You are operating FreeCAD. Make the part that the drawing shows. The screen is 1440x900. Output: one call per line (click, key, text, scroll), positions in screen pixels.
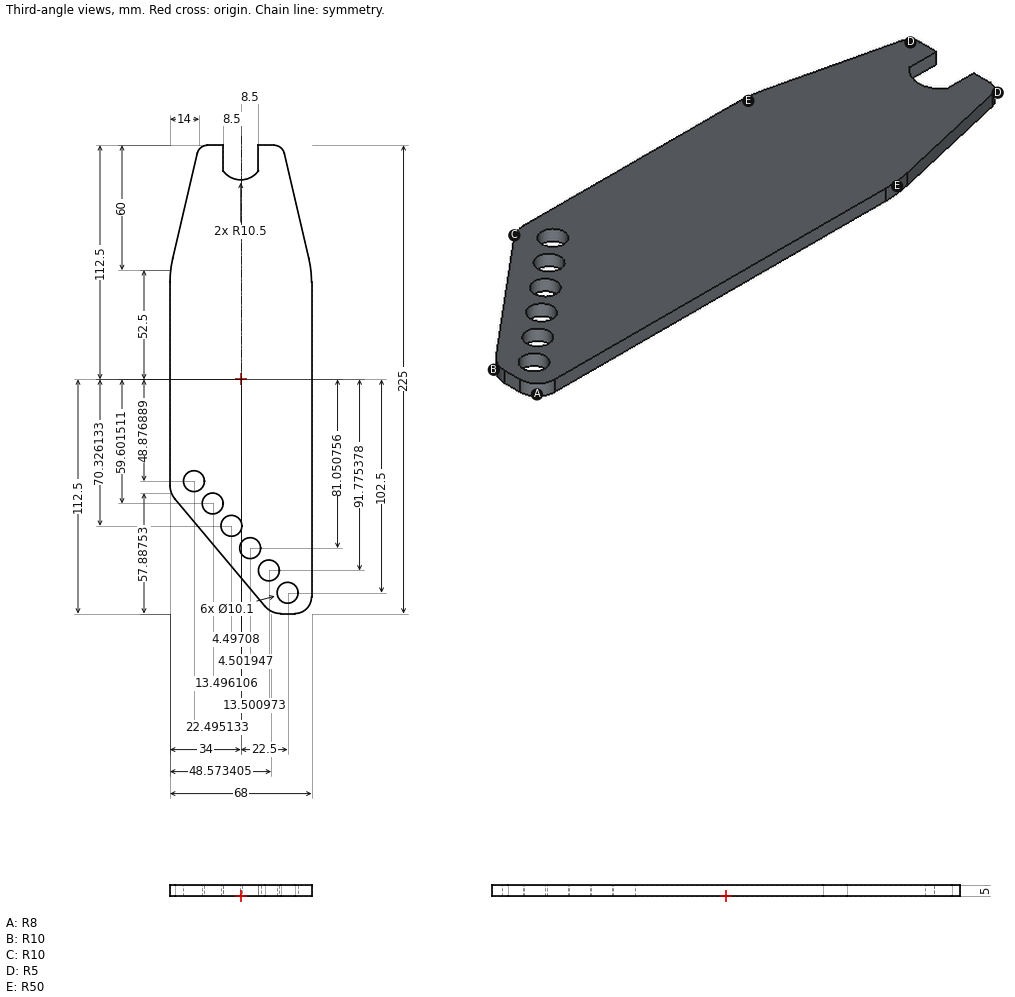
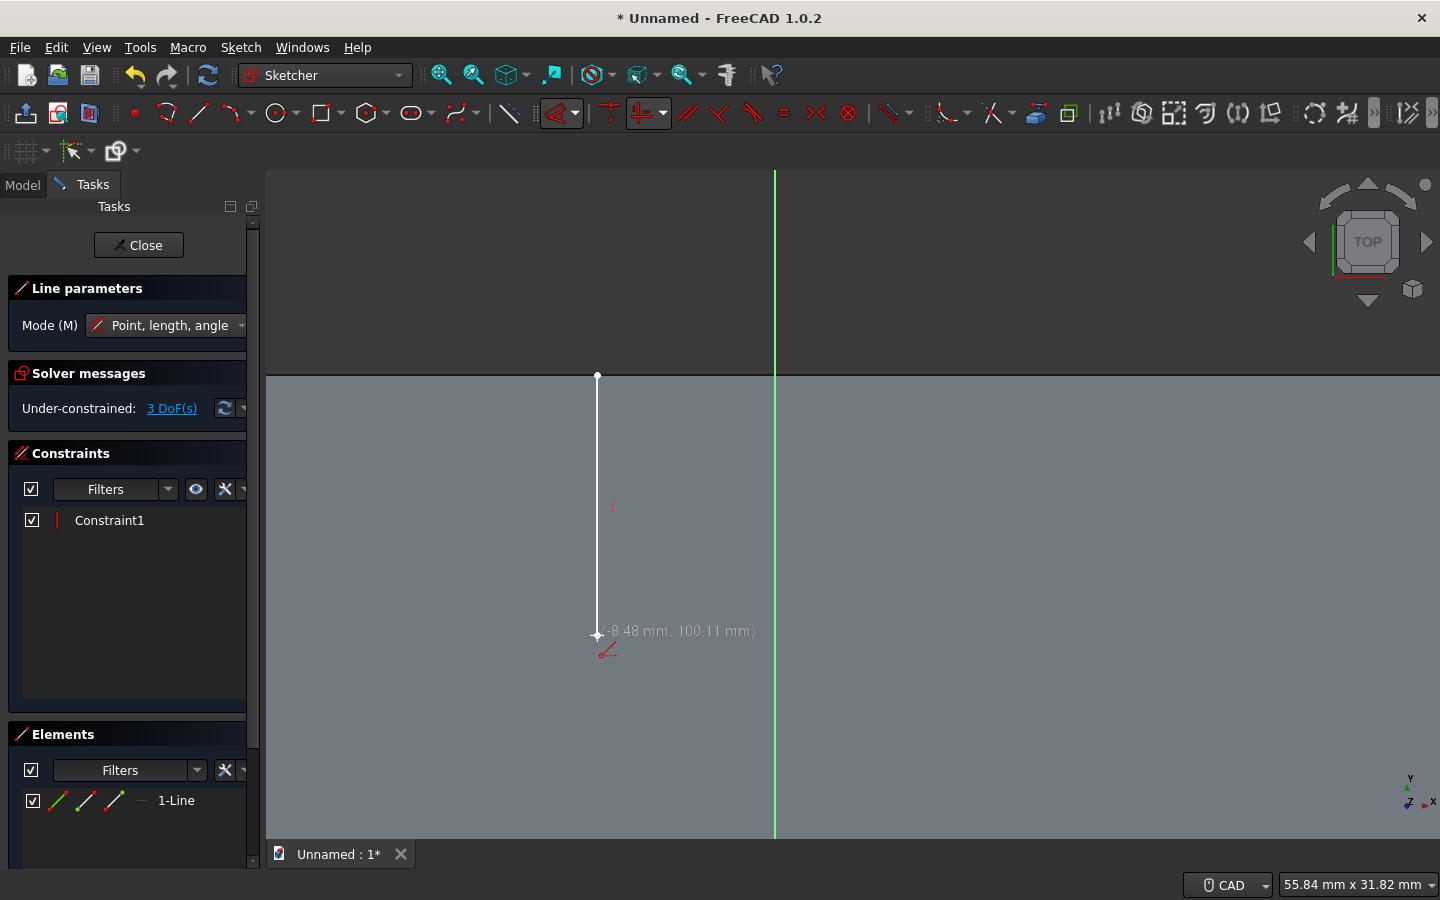
click(954, 635)
click(954, 375)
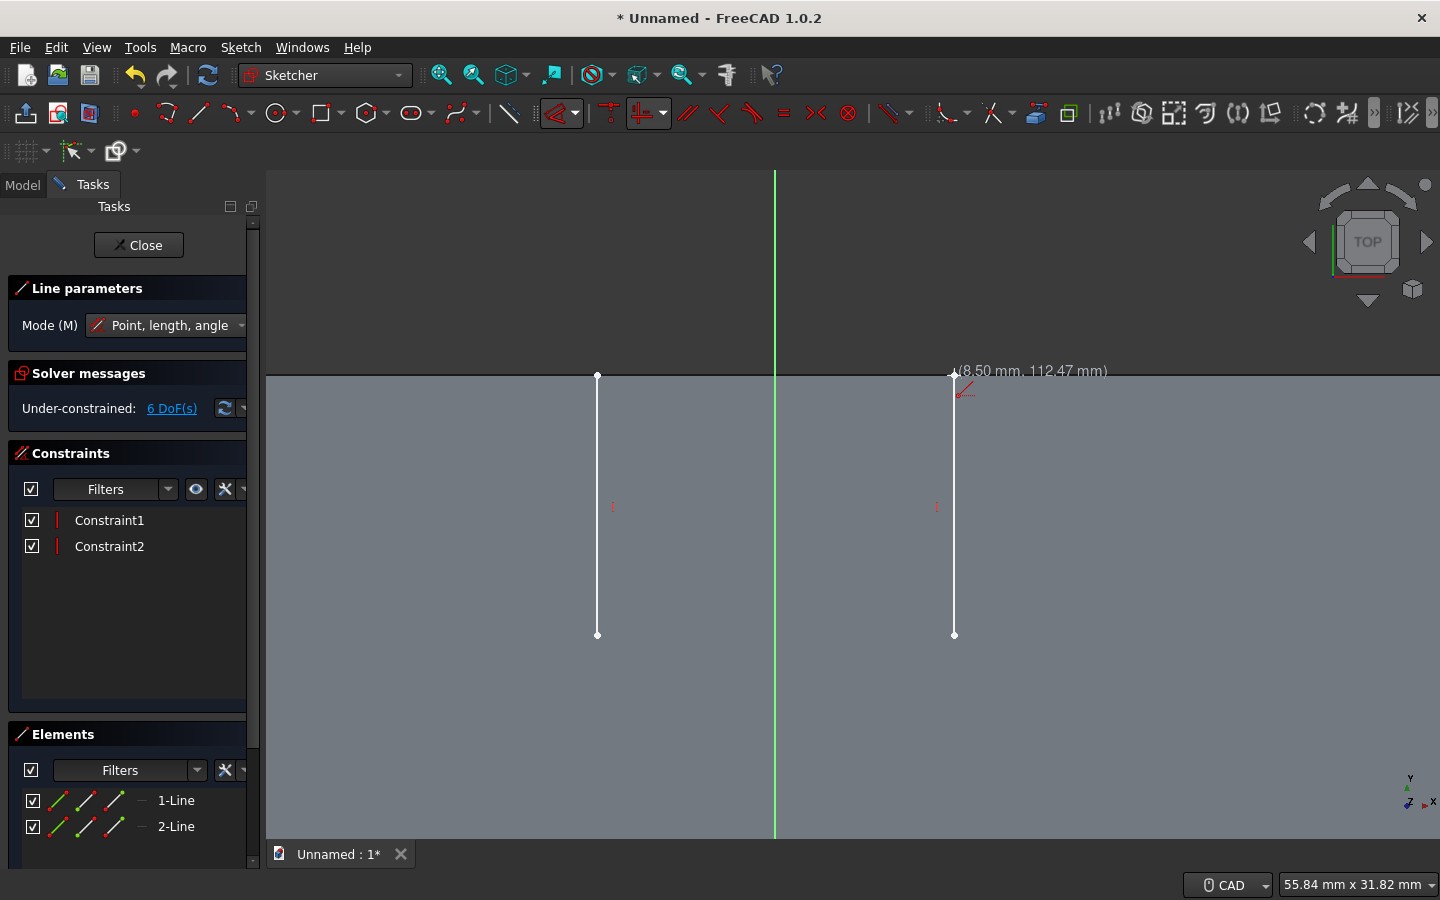
key(g)
key(3)
key(a)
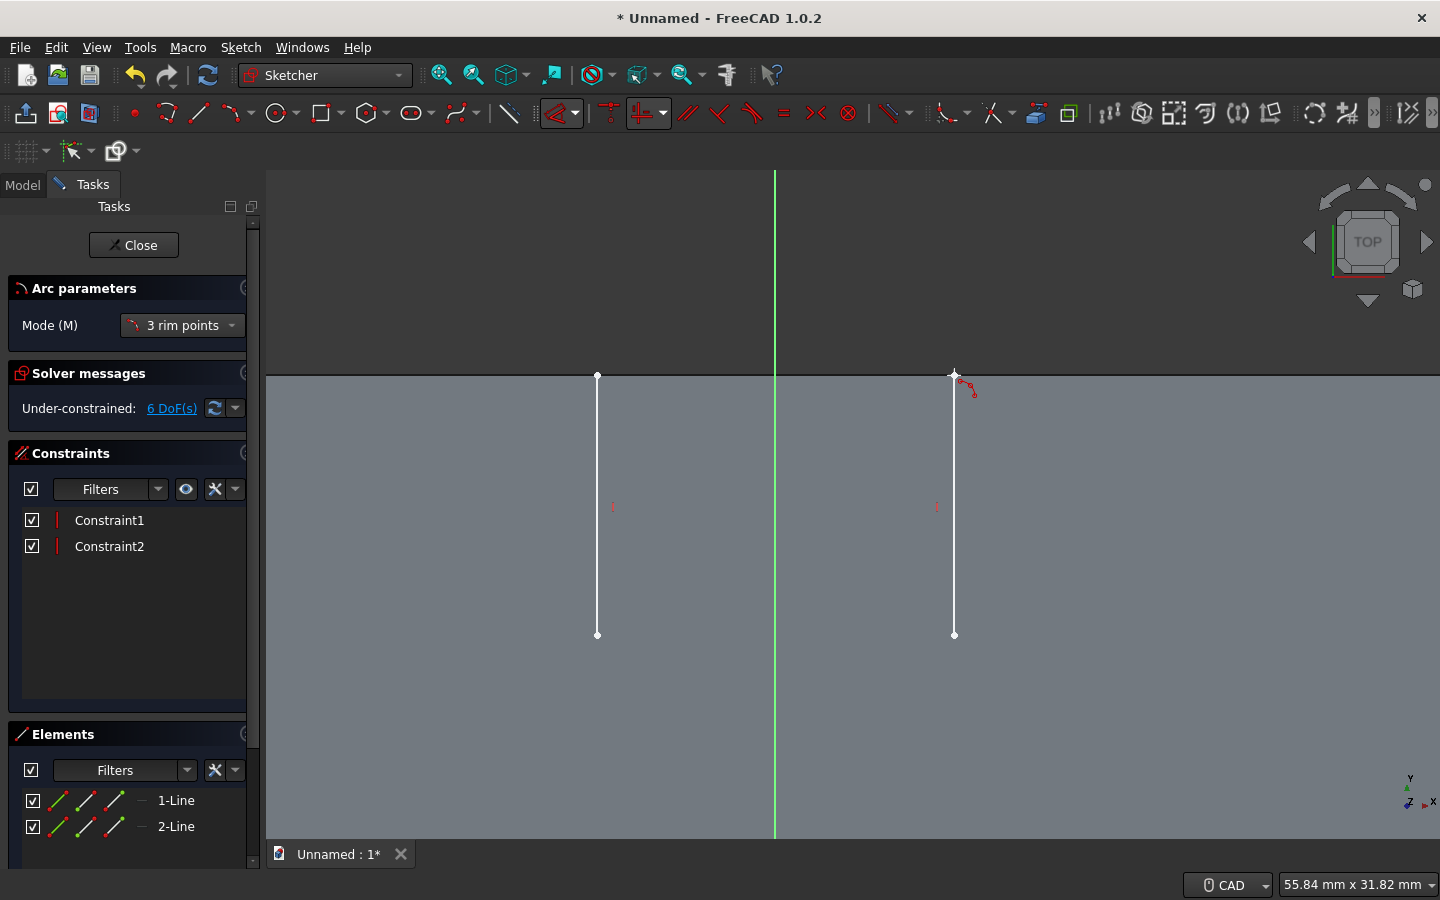
click(597, 636)
click(954, 636)
click(734, 722)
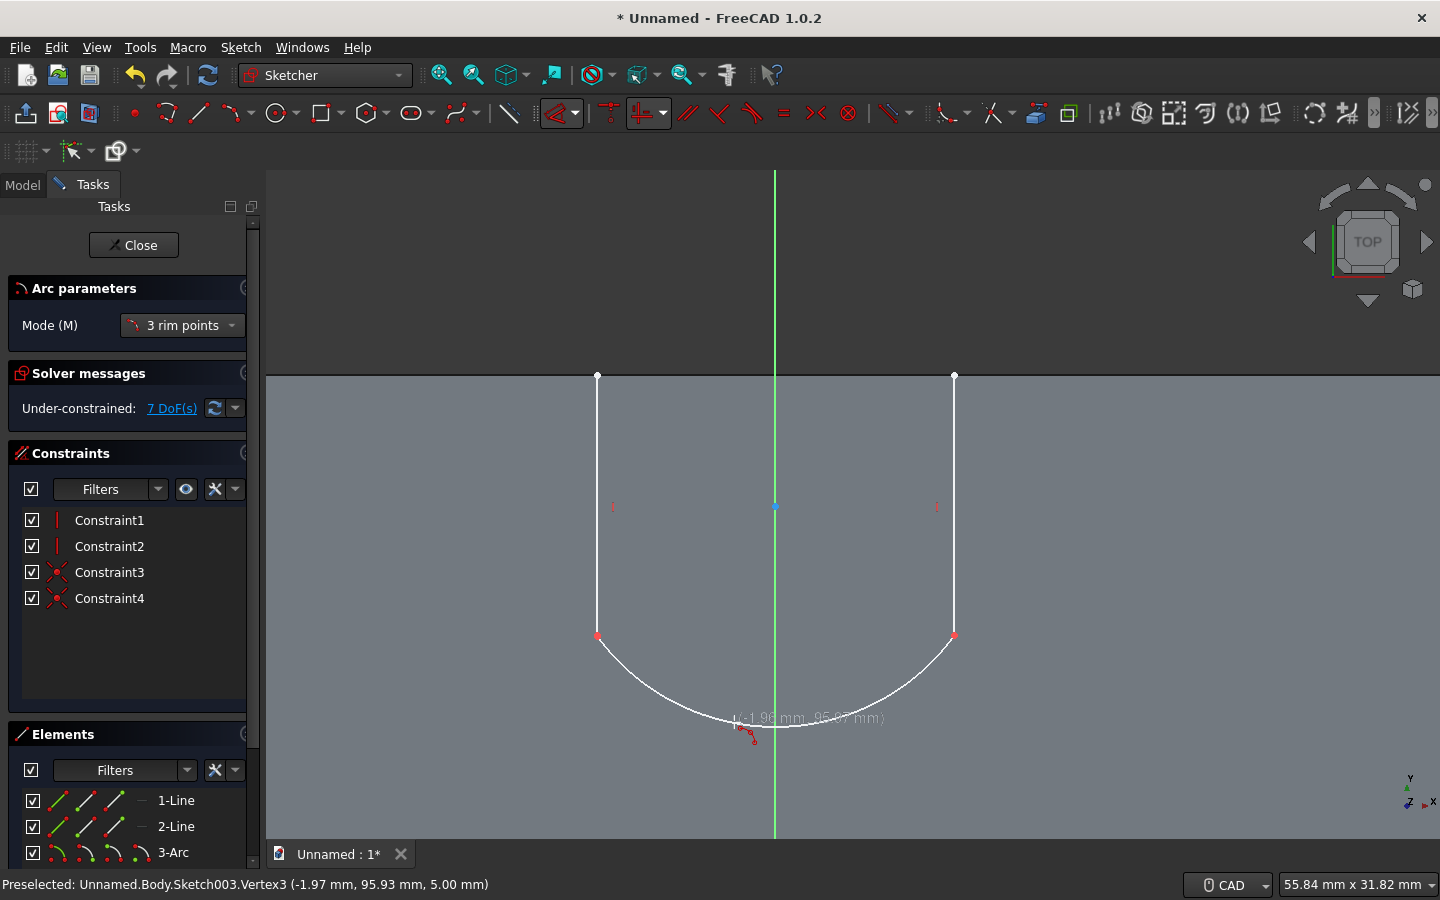
click(954, 376)
click(597, 376)
click(817, 288)
key(Escape)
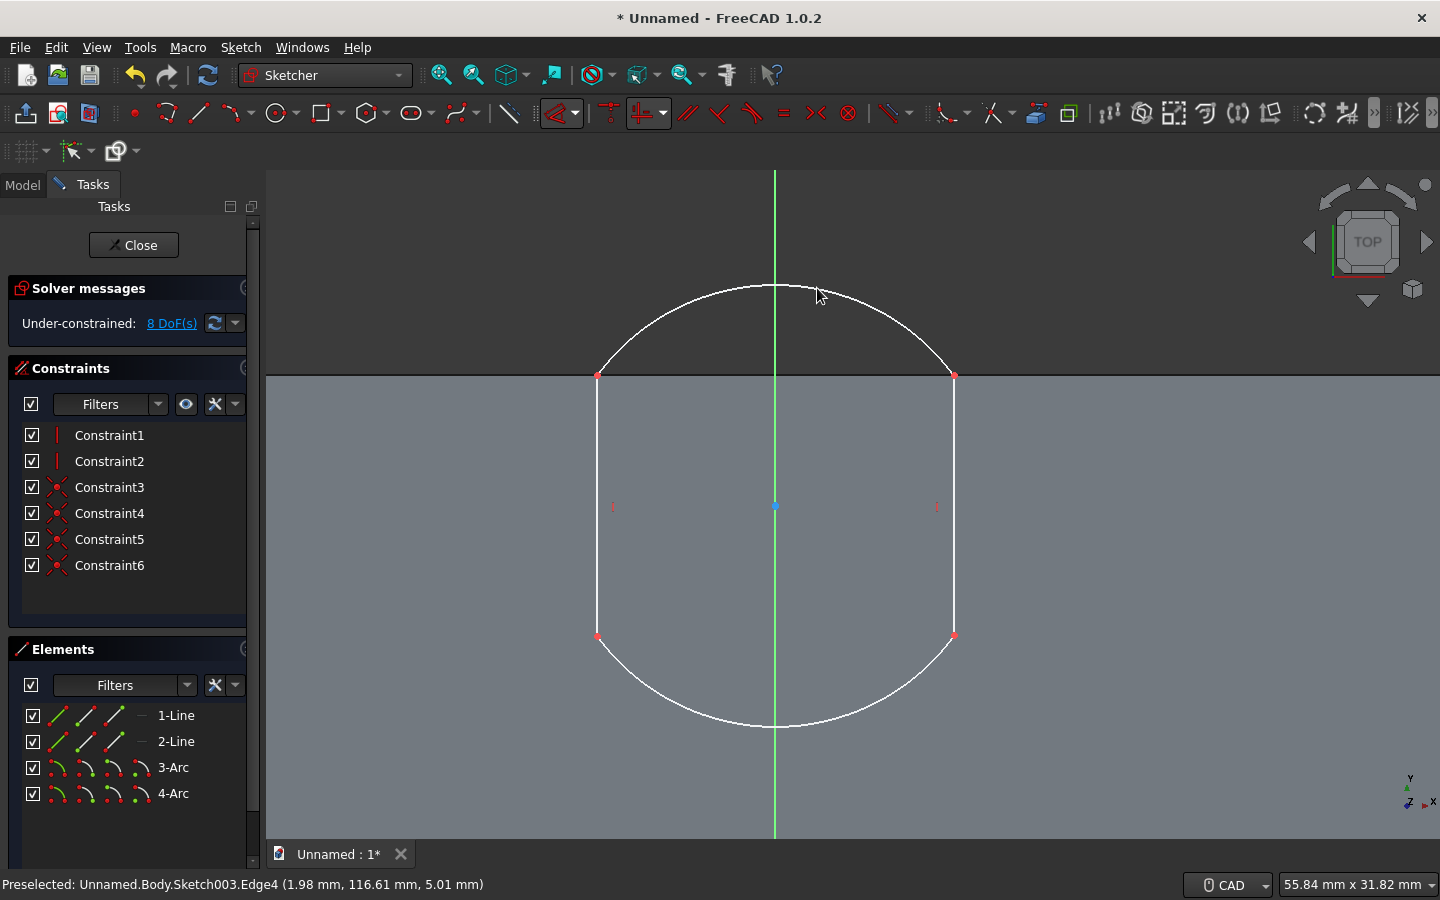
click(694, 711)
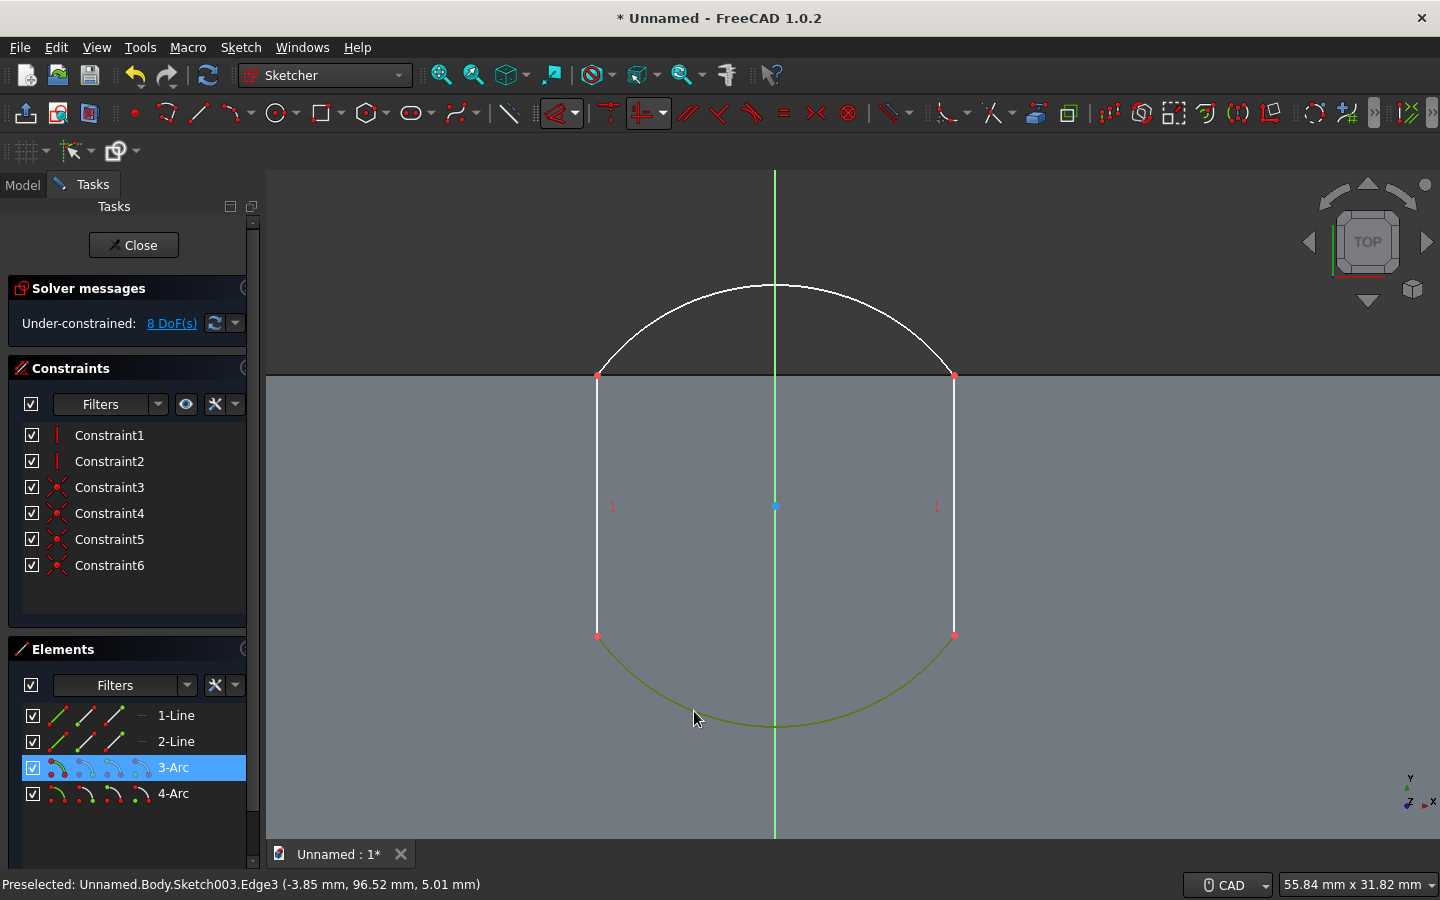
click(857, 301)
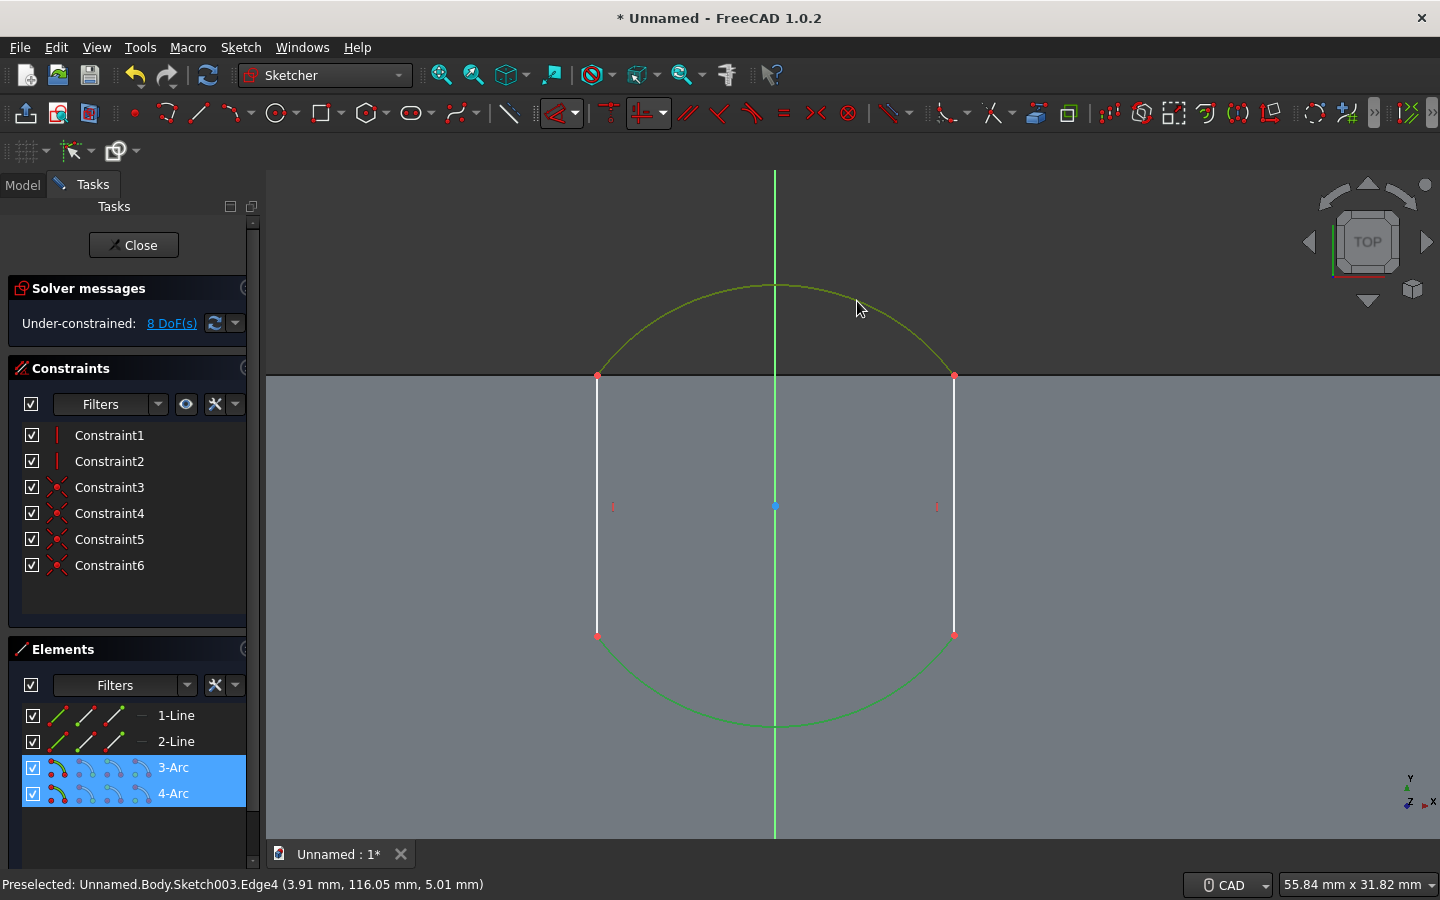
key(c)